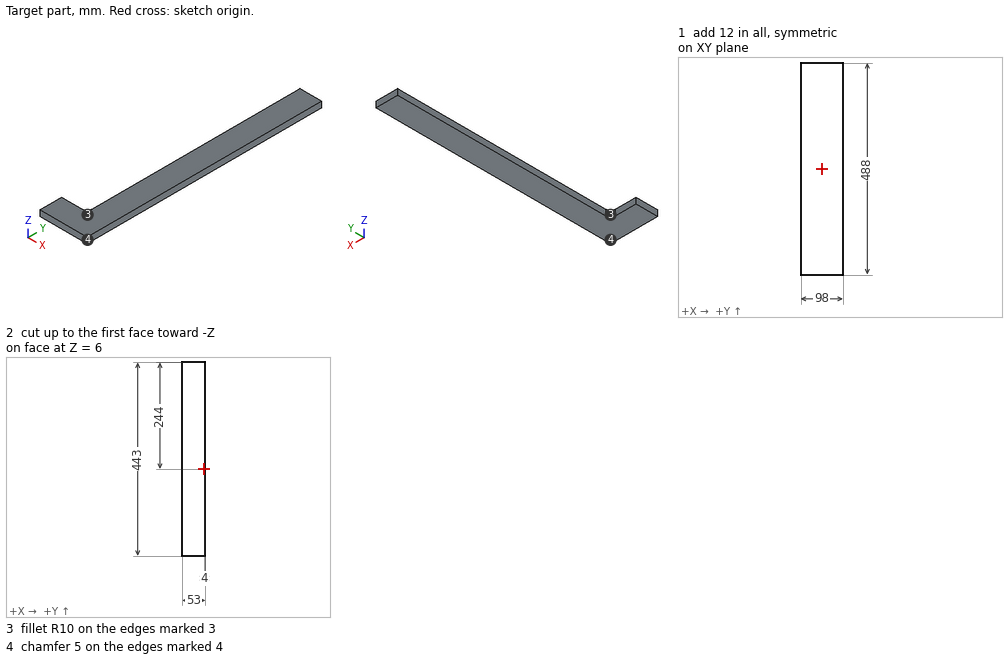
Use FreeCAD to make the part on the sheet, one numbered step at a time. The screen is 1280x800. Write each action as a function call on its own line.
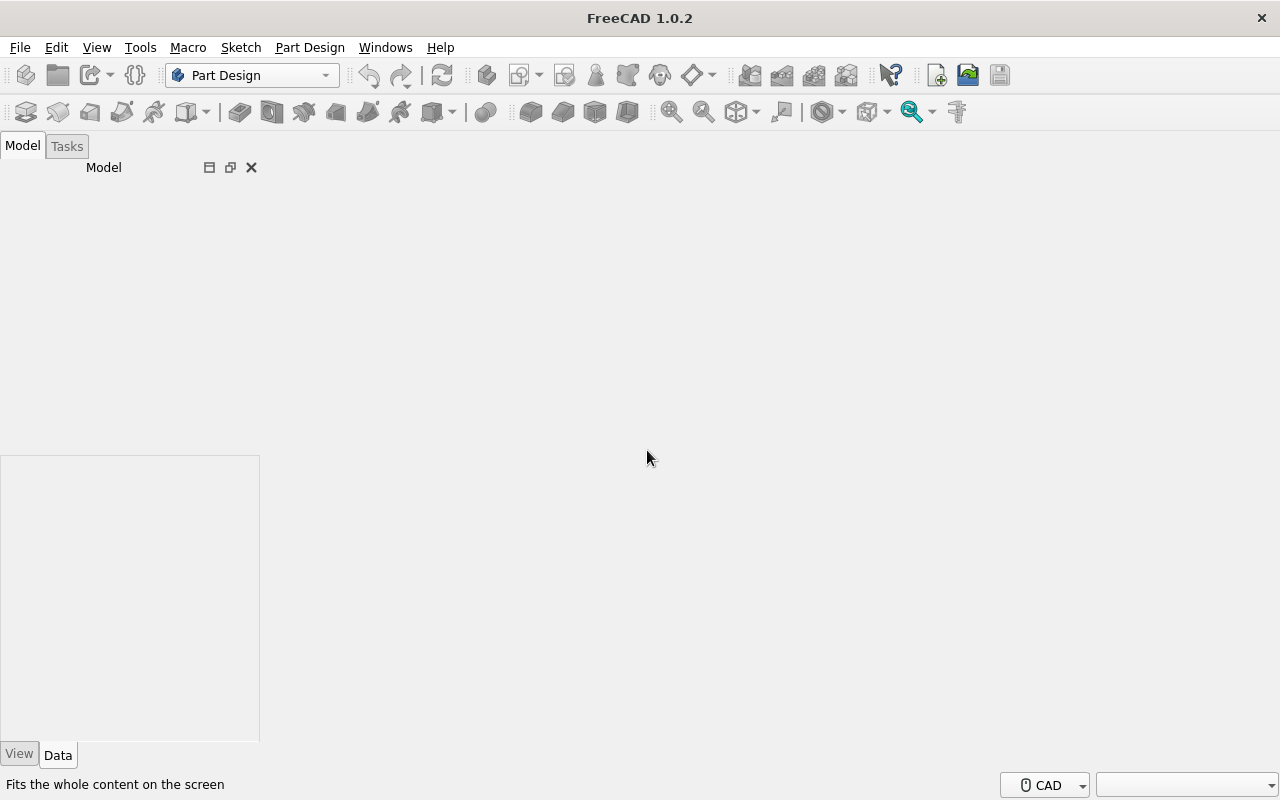
key(ctrl+n)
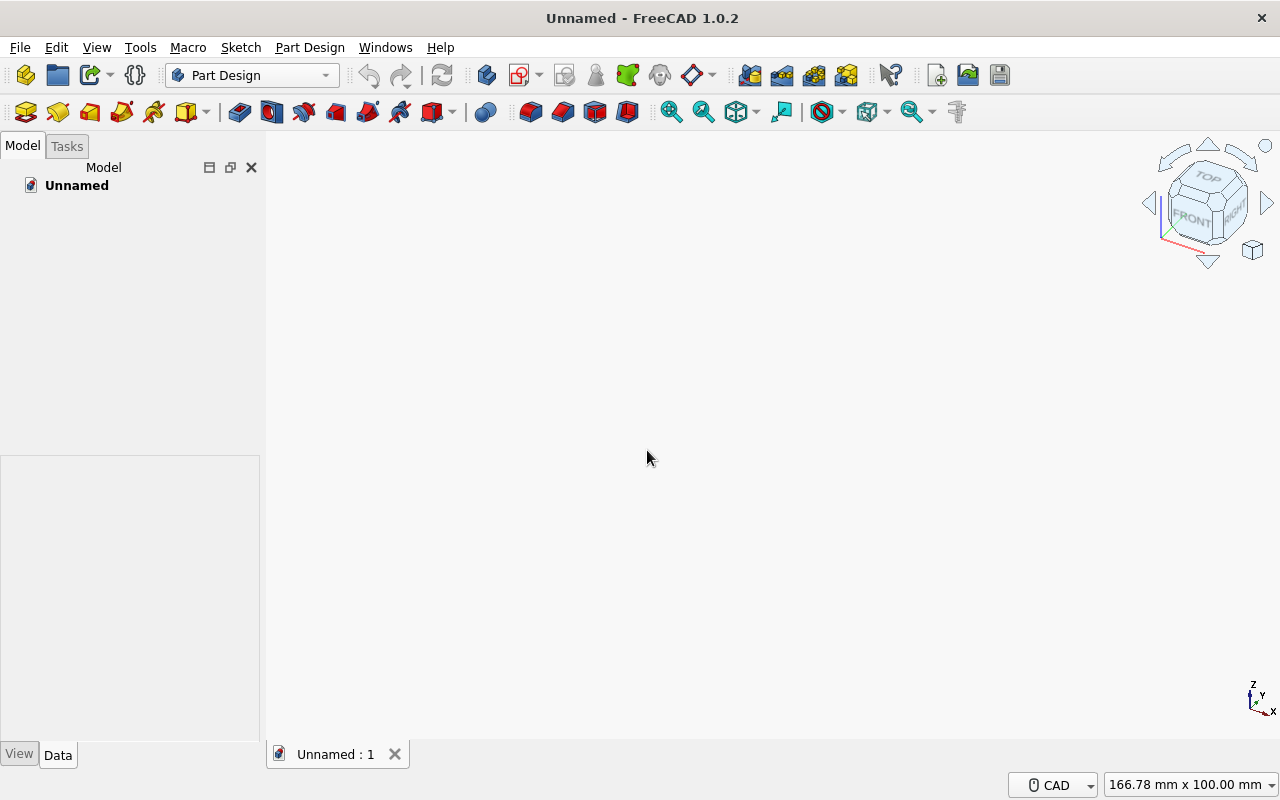
click(520, 76)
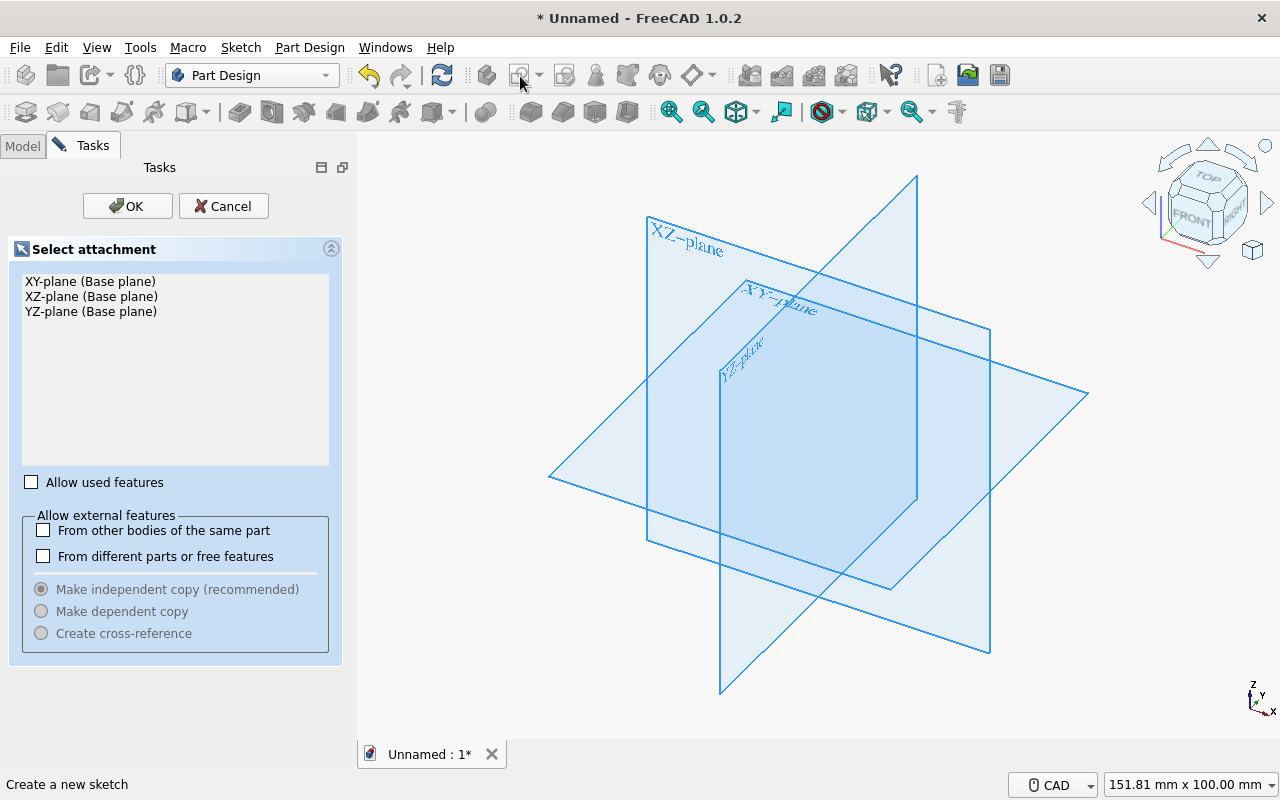
click(82, 282)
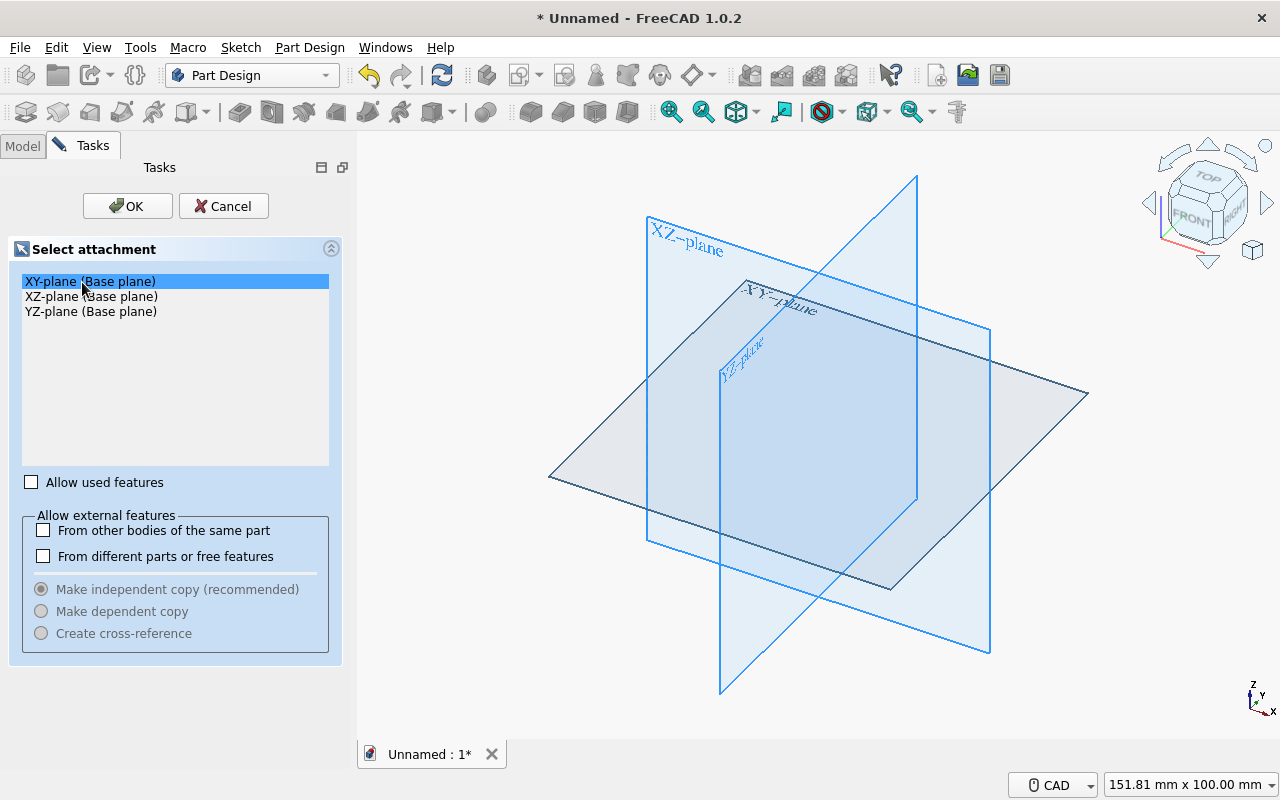
click(128, 206)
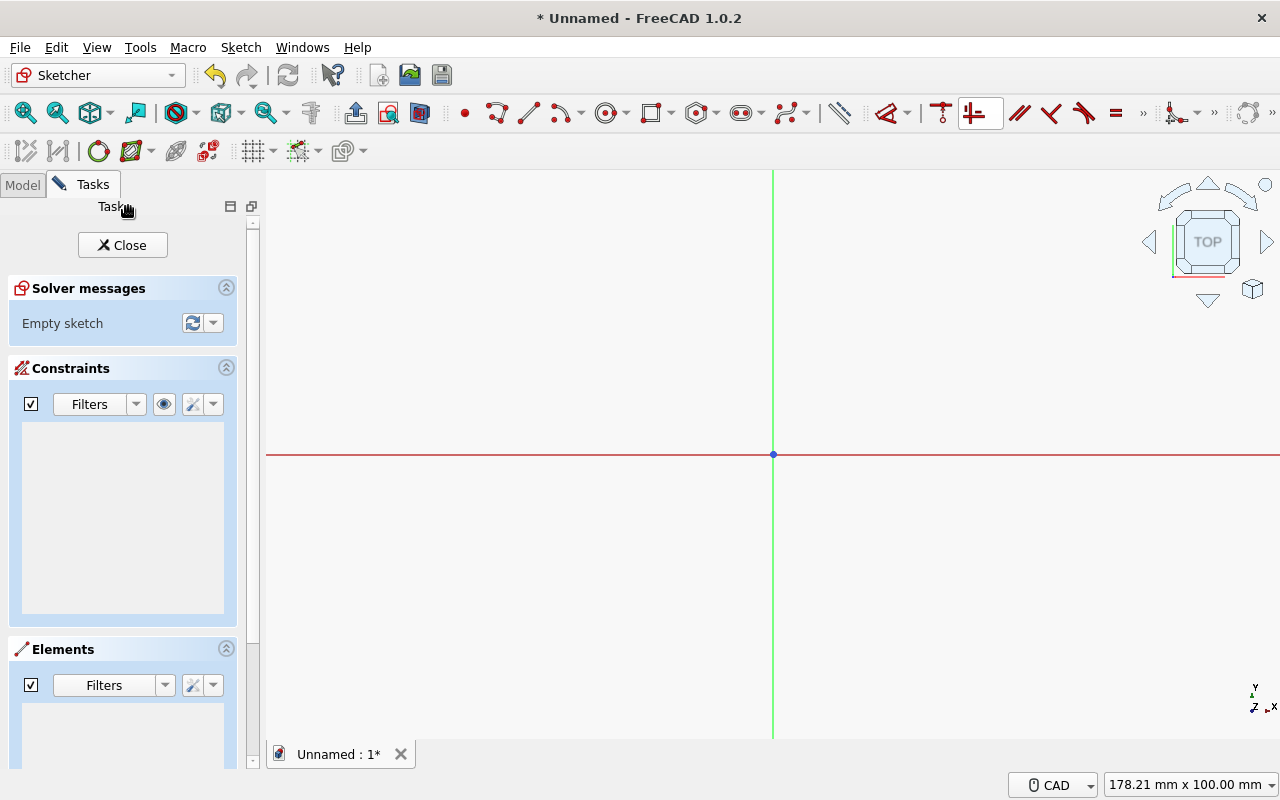
scroll(694, 454, down, 10)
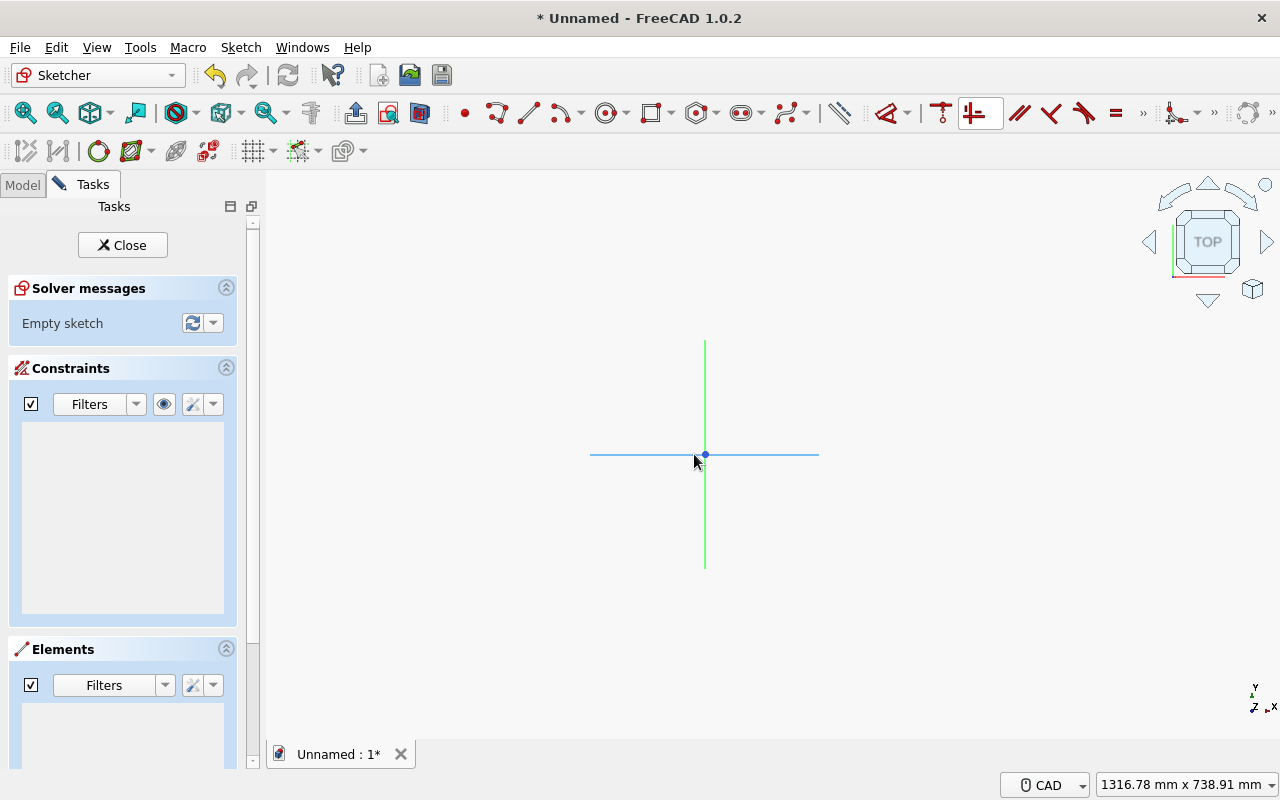
key(g)
key(v)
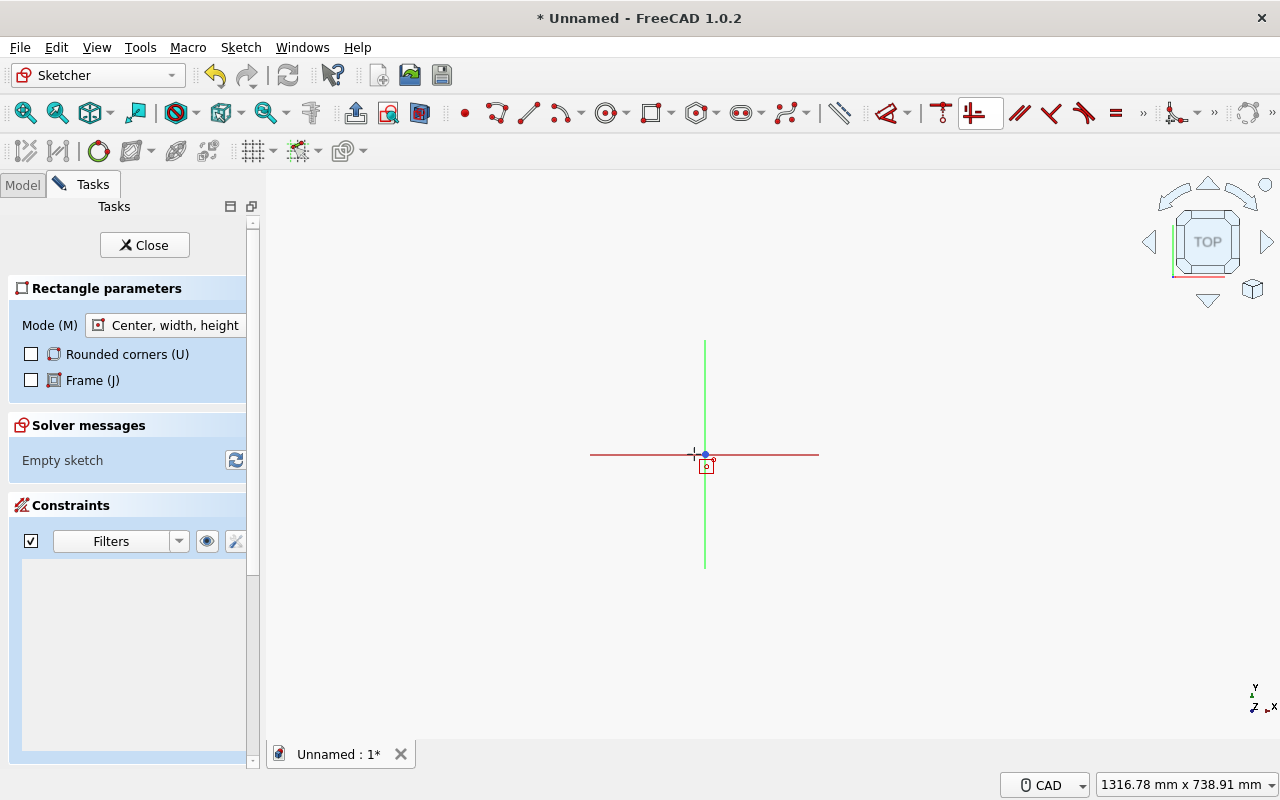
click(705, 454)
click(743, 267)
key(Escape)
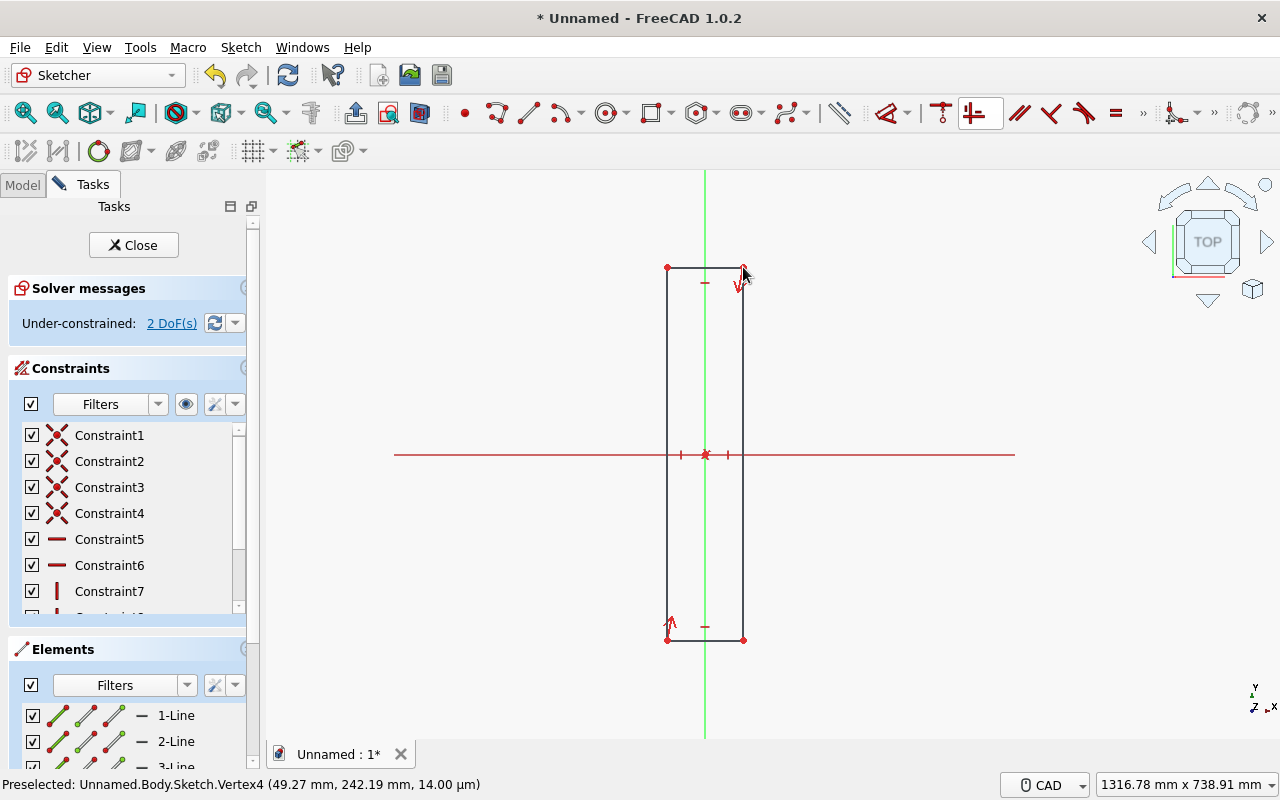
click(690, 641)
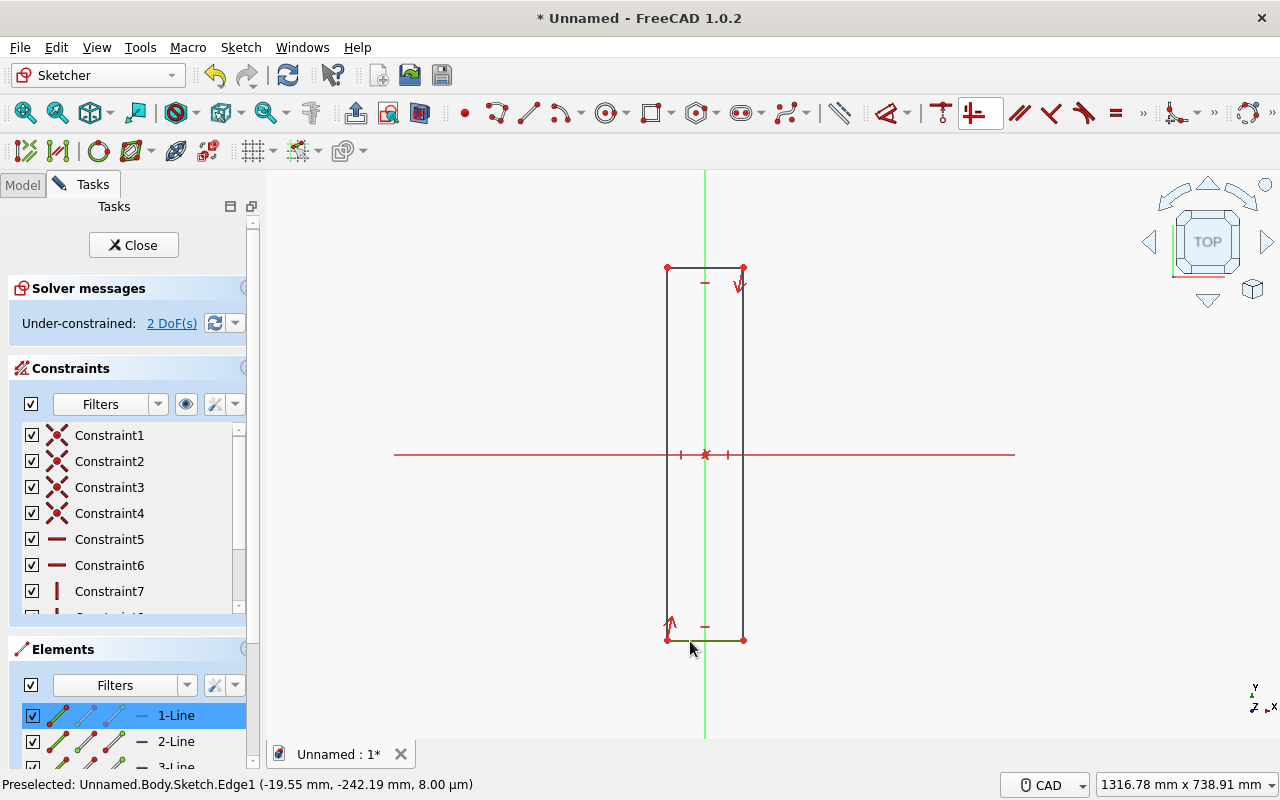
key(l)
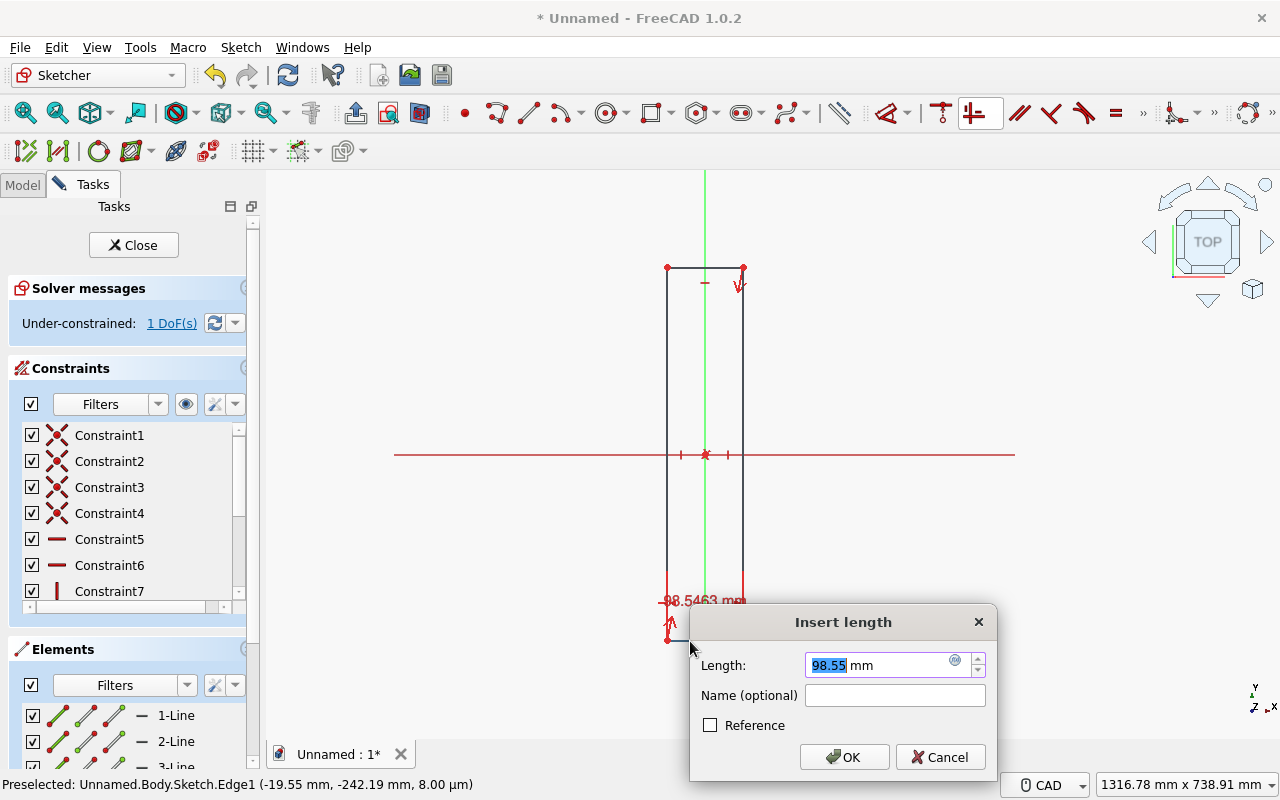
text(98)
key(Return)